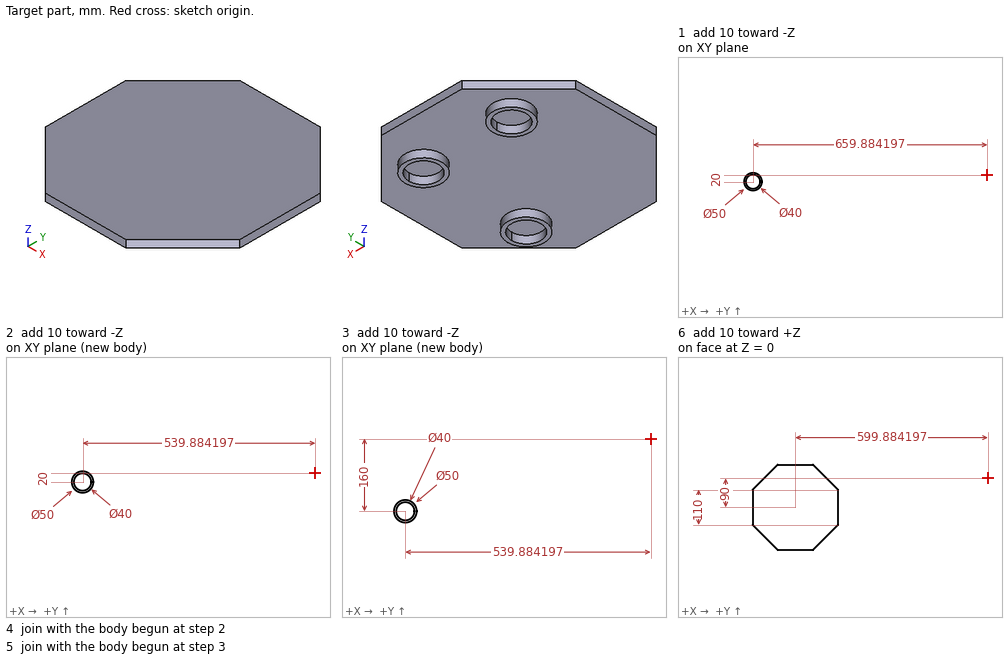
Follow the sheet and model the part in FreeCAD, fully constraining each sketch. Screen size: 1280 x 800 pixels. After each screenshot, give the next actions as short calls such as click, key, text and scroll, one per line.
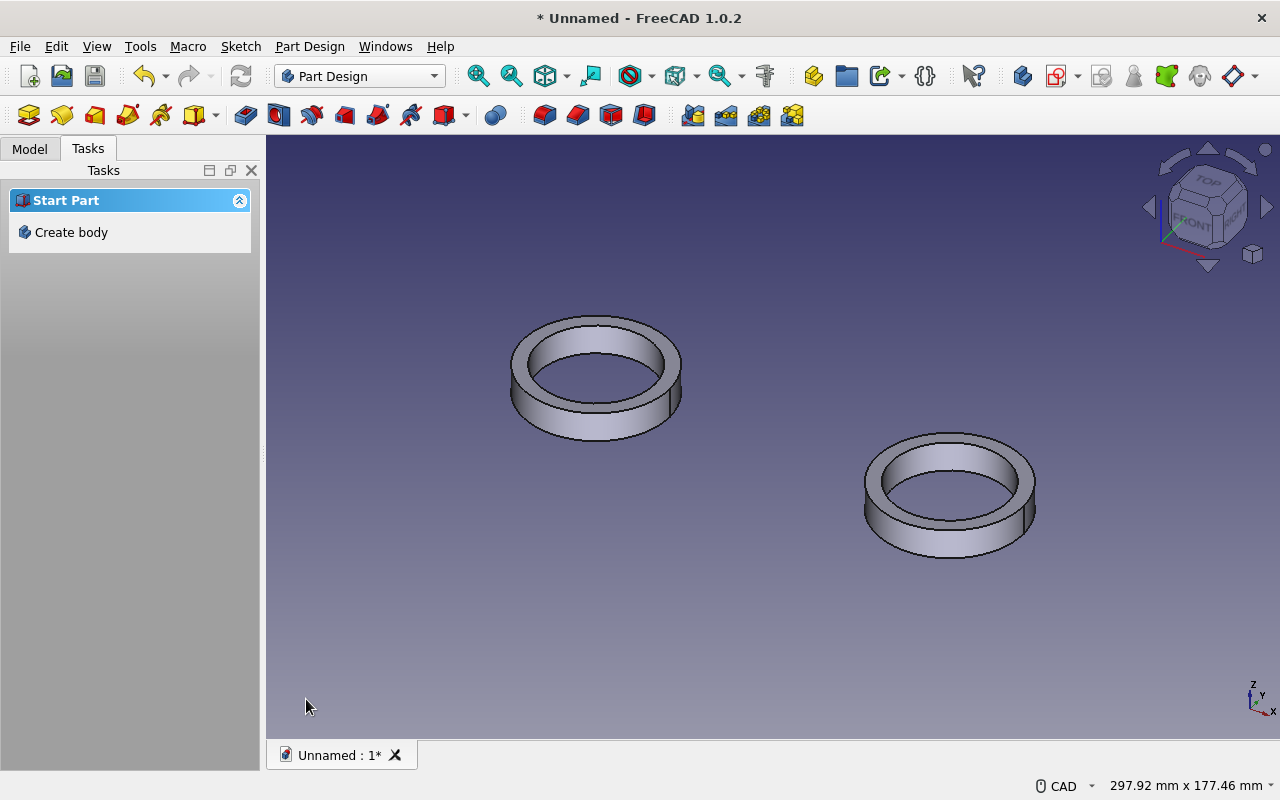
click(1056, 76)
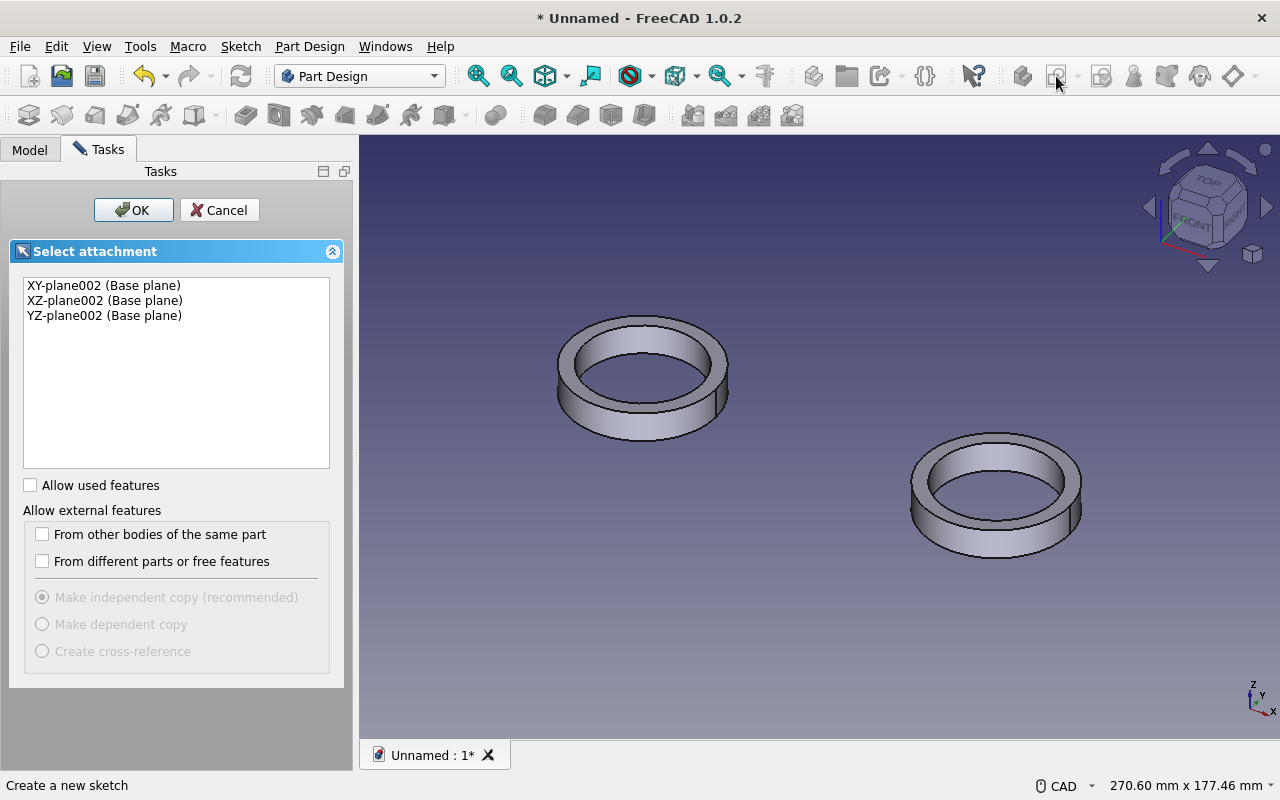
click(84, 286)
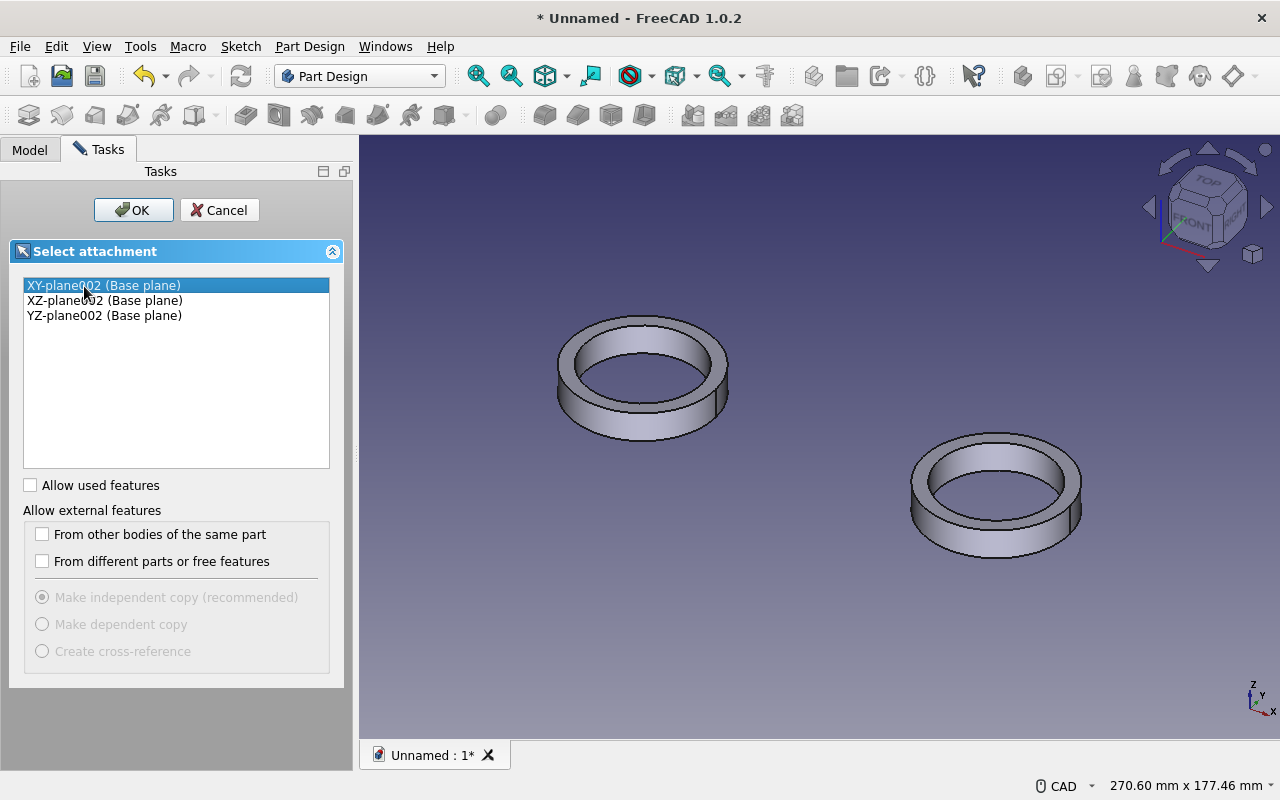
click(134, 210)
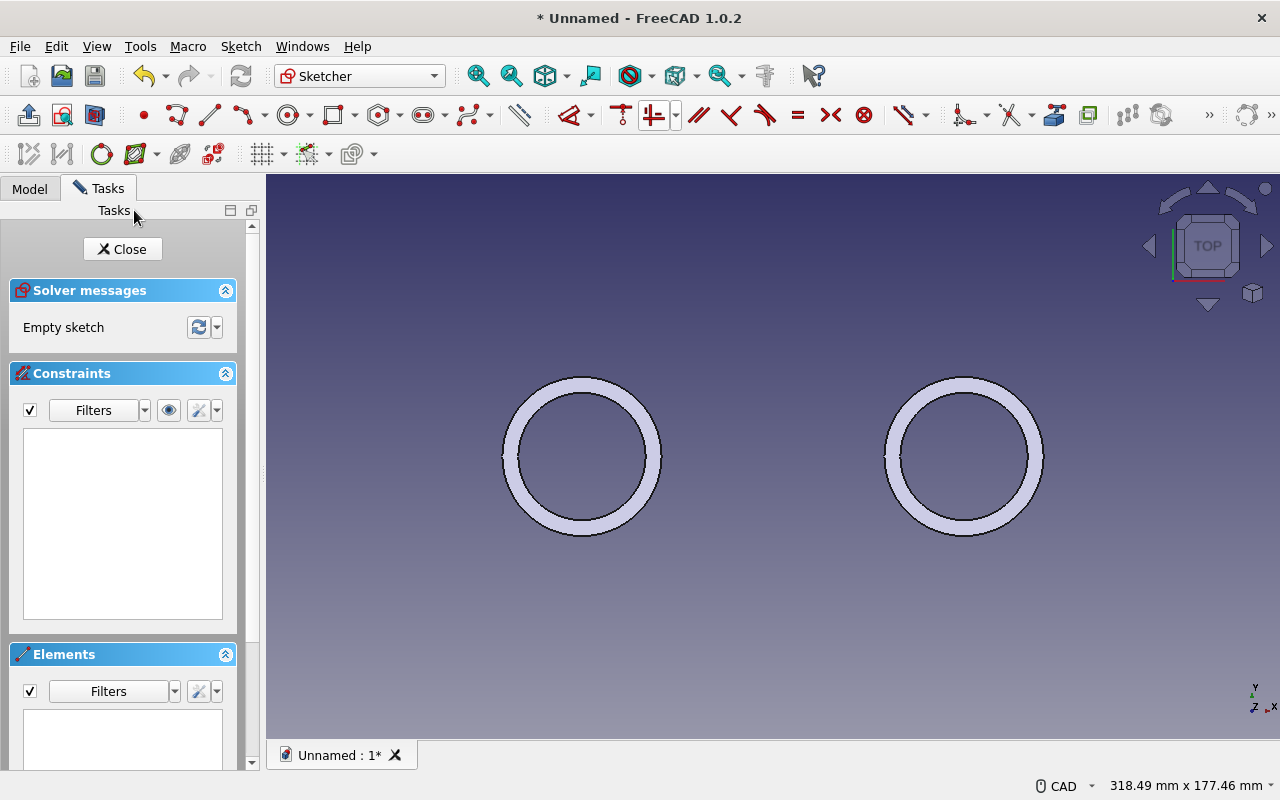
scroll(704, 456, down, 5)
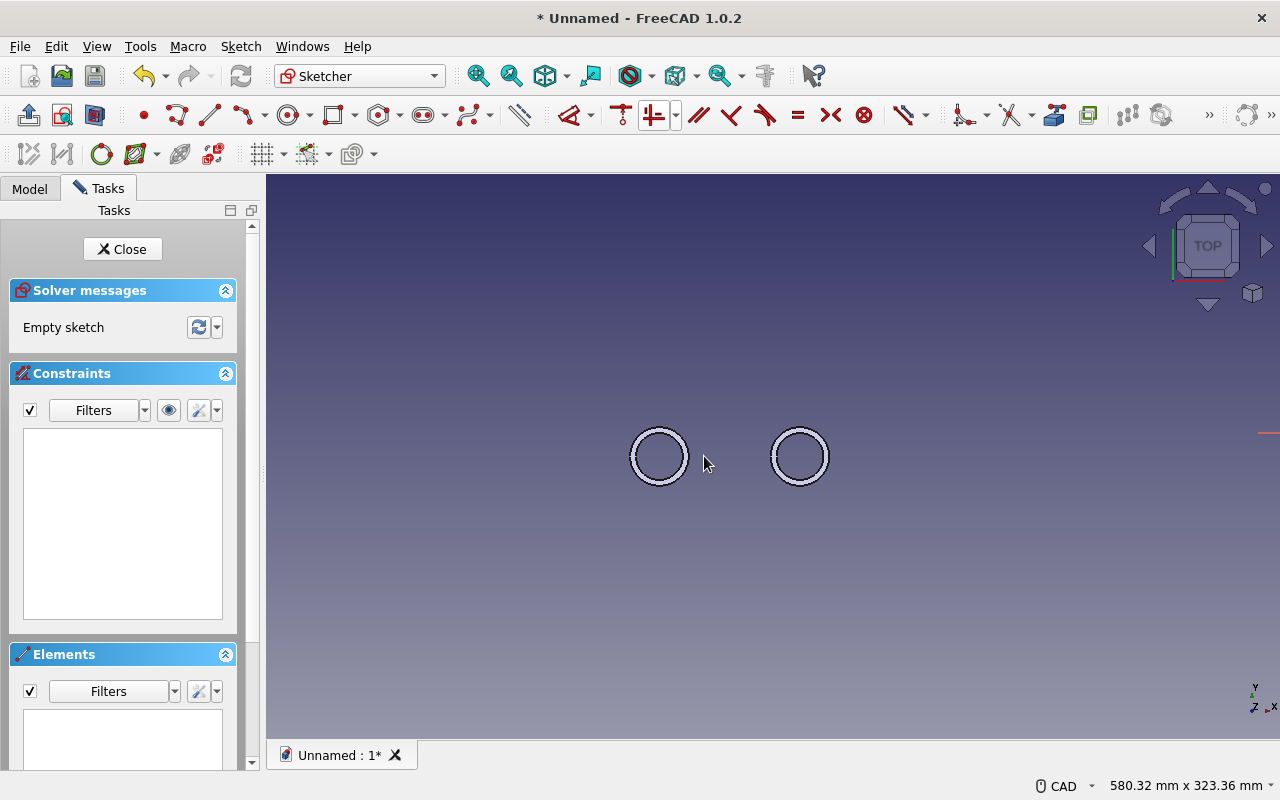
scroll(819, 653, up, 9)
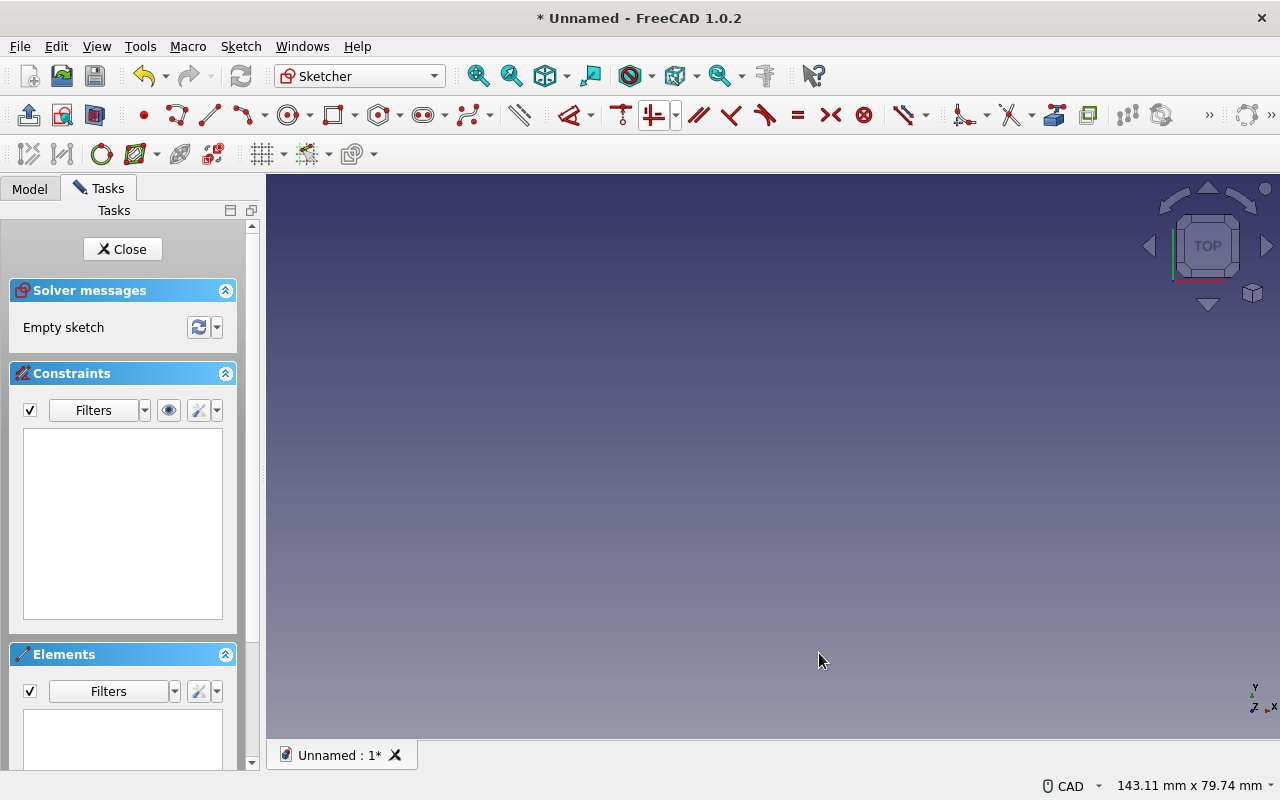
key(g)
key(c)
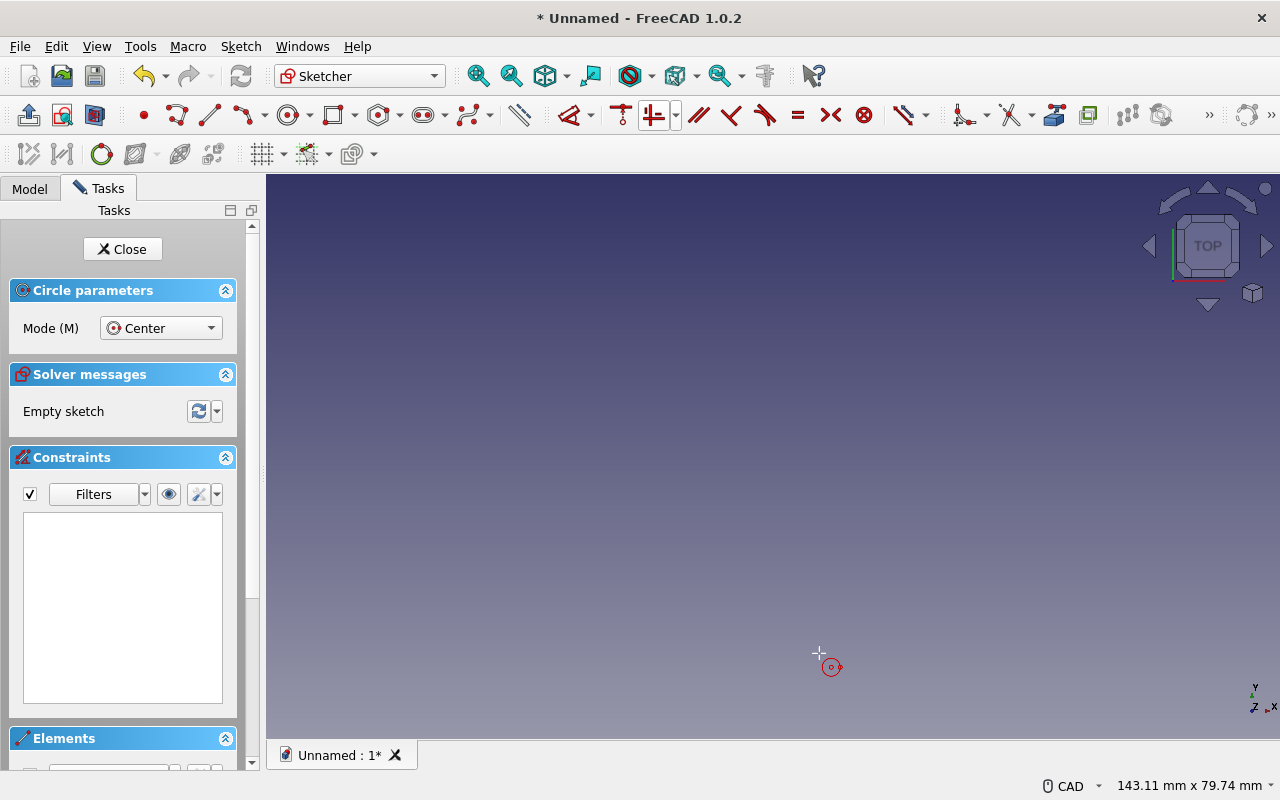
click(701, 452)
move(826, 327)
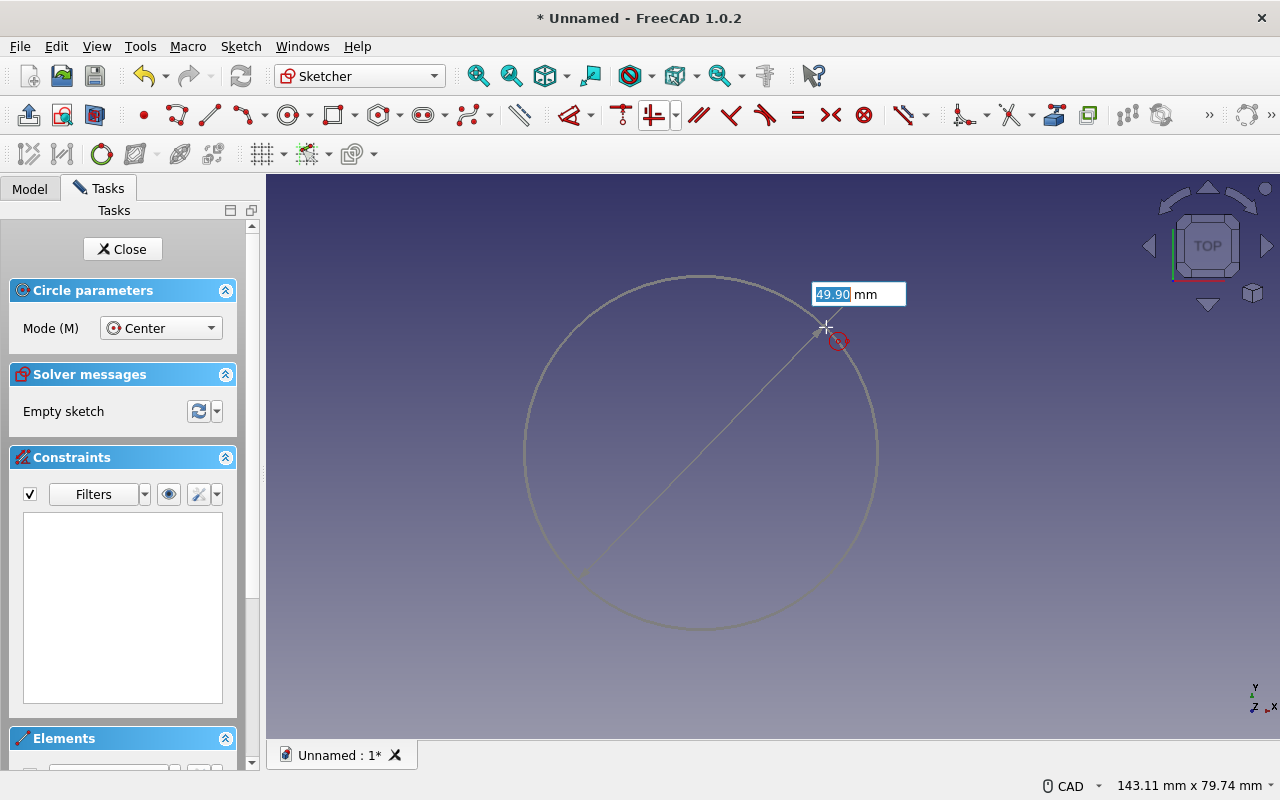
text(50)
key(Return)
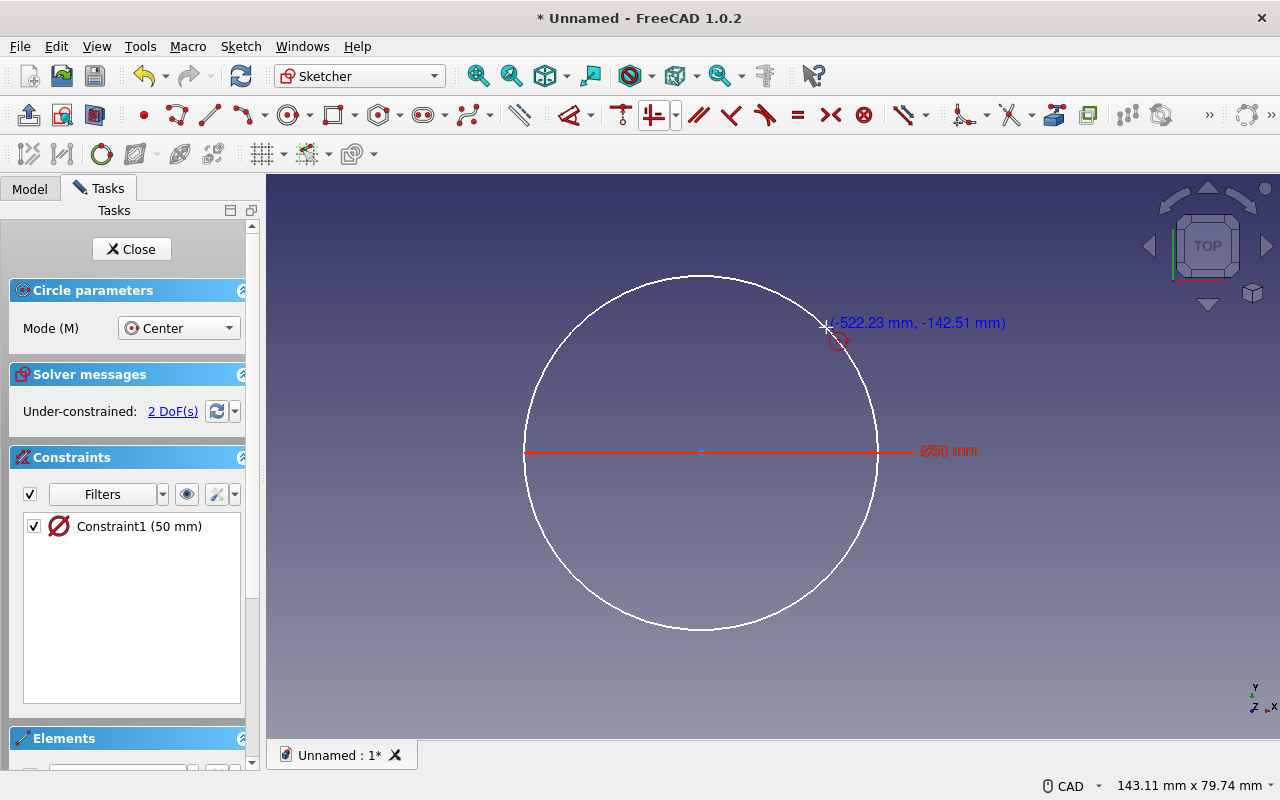
click(701, 453)
move(801, 352)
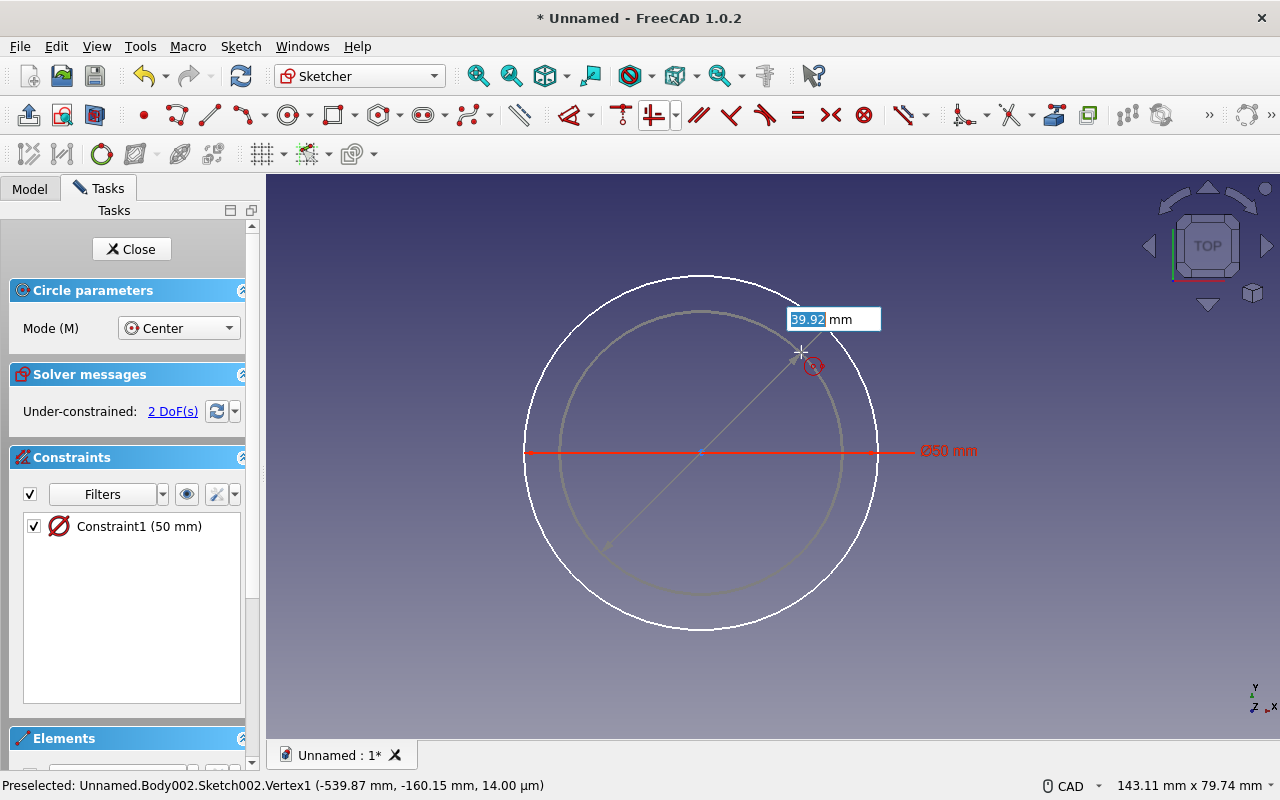
text(40)
key(Return)
key(Escape)